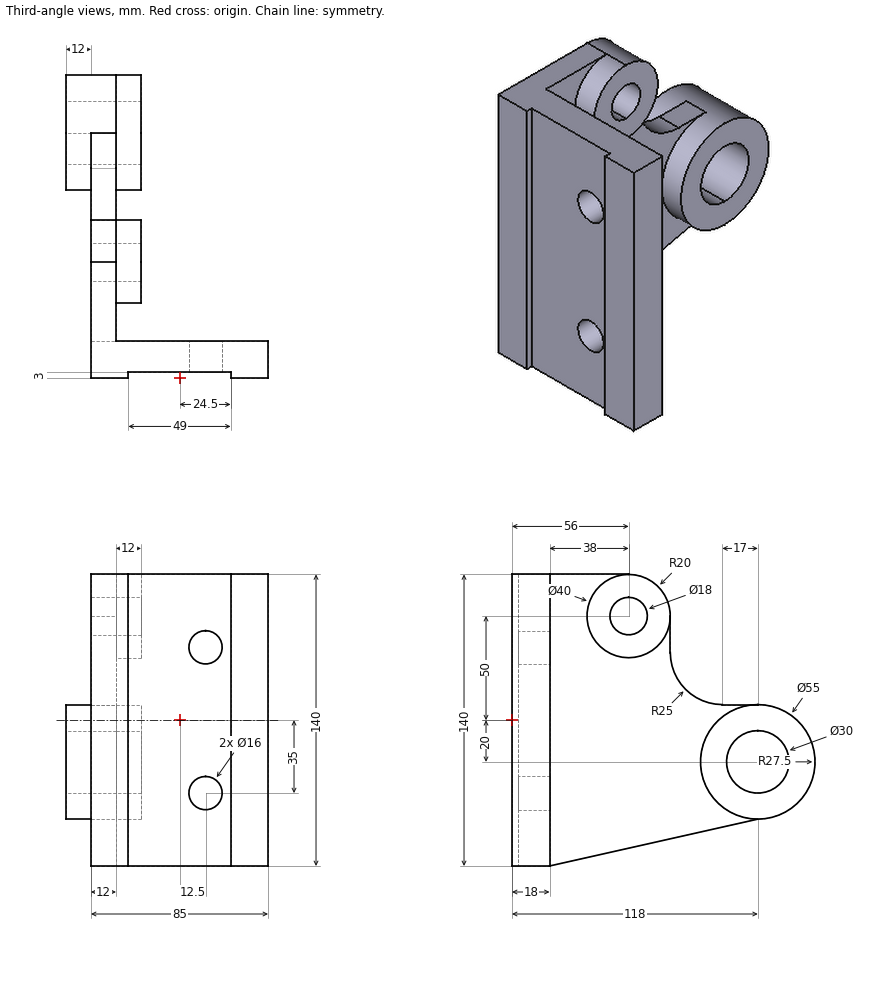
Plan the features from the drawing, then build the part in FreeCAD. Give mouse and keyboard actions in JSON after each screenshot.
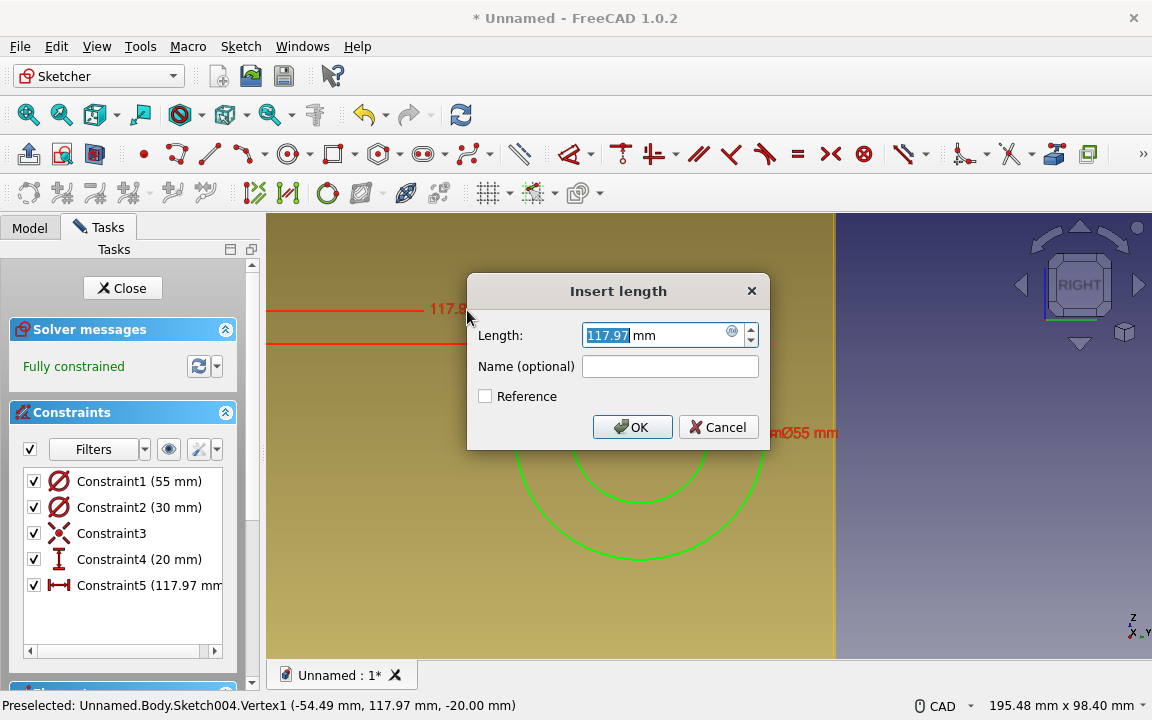
{"action": "type", "text": "118"}
{"action": "key", "text": "Return"}
{"action": "key", "text": "Escape"}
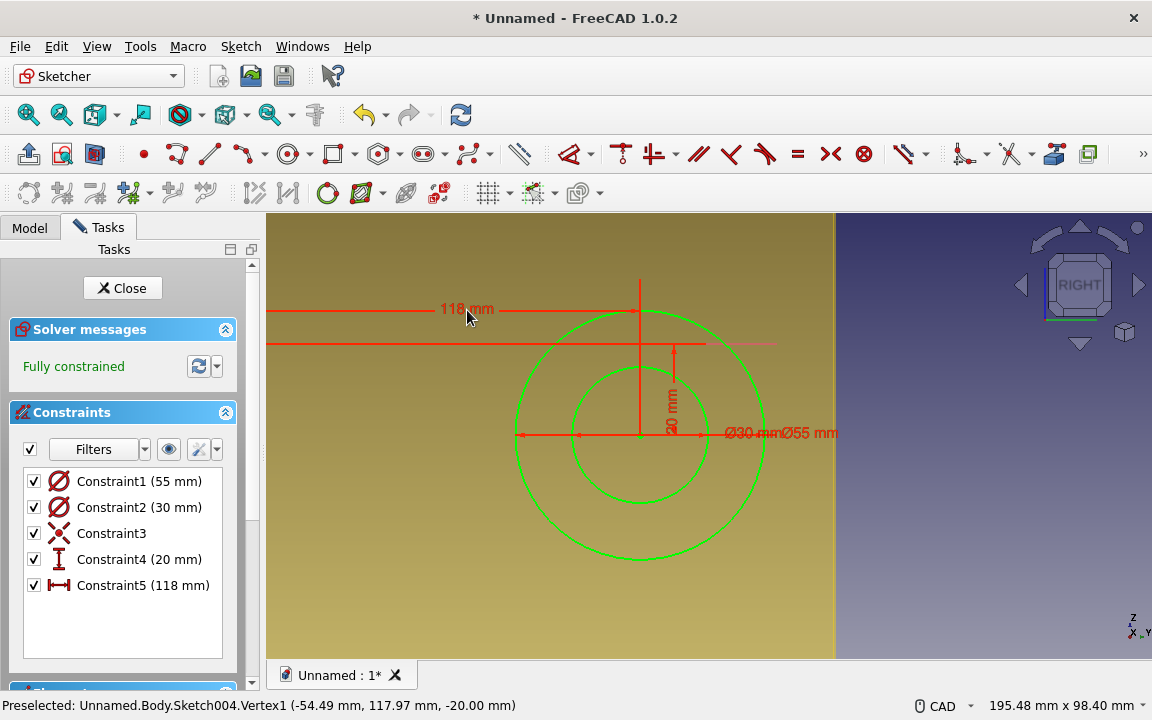
{"action": "left_click", "coordinate": [123, 288]}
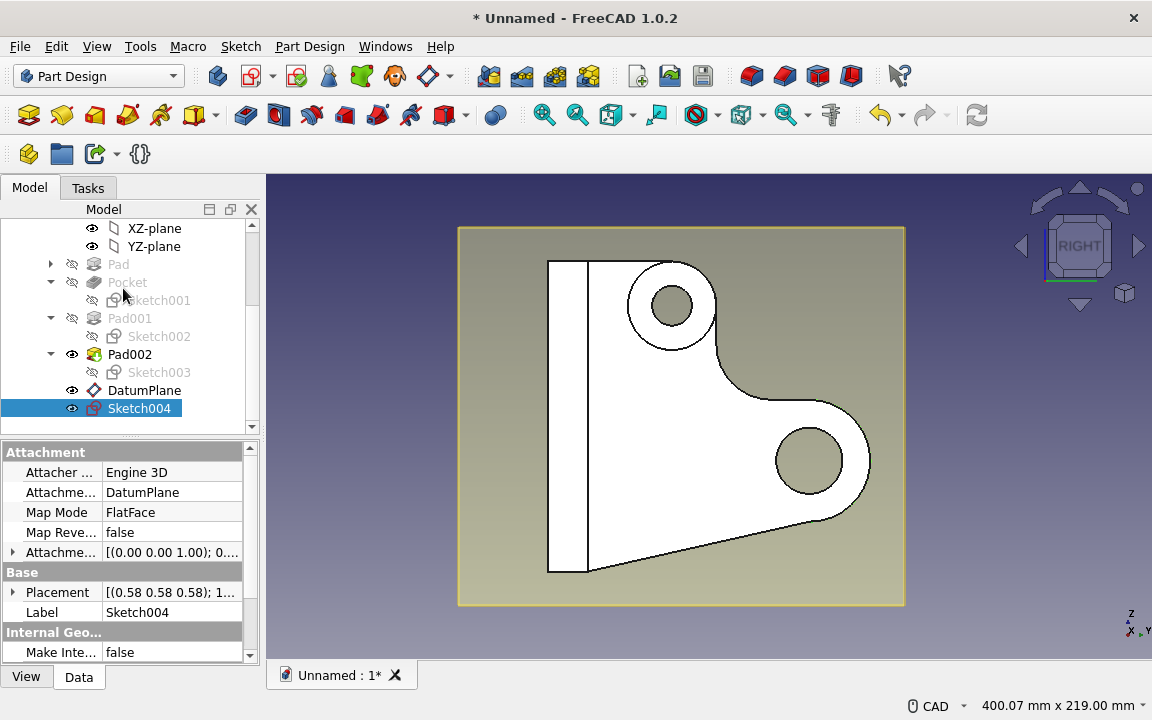
{"action": "left_click", "coordinate": [29, 116]}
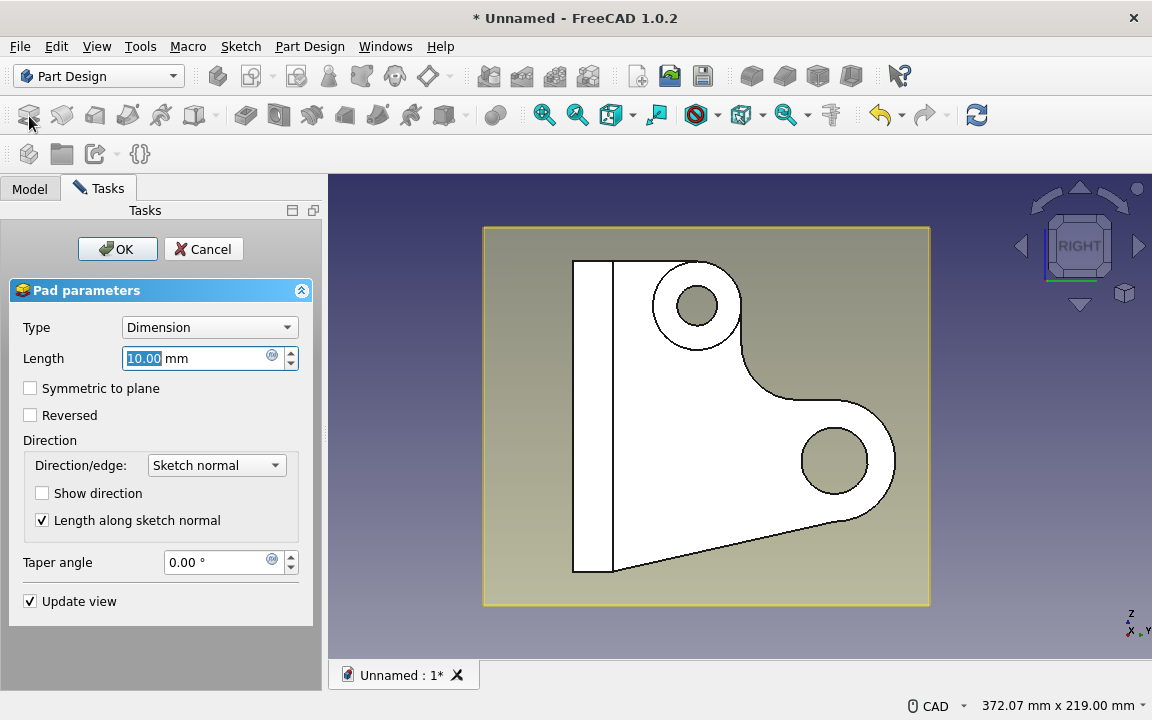
{"action": "type", "text": "12"}
{"action": "key", "text": "Tab"}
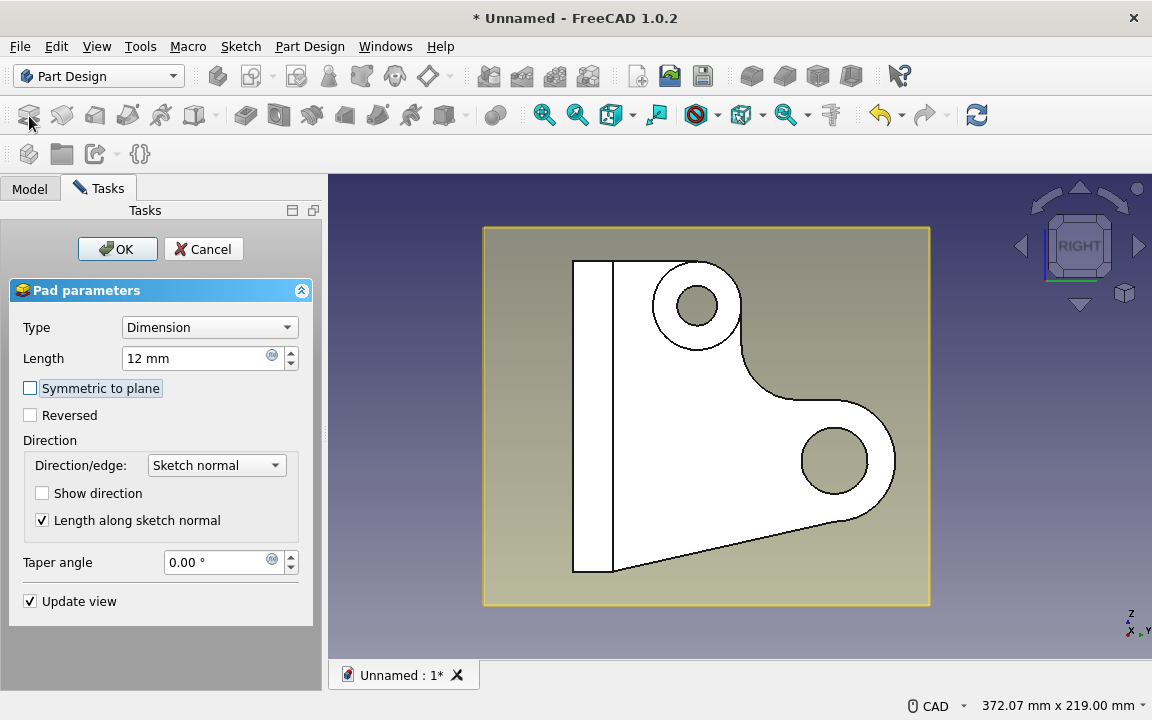
{"action": "left_click", "coordinate": [118, 249]}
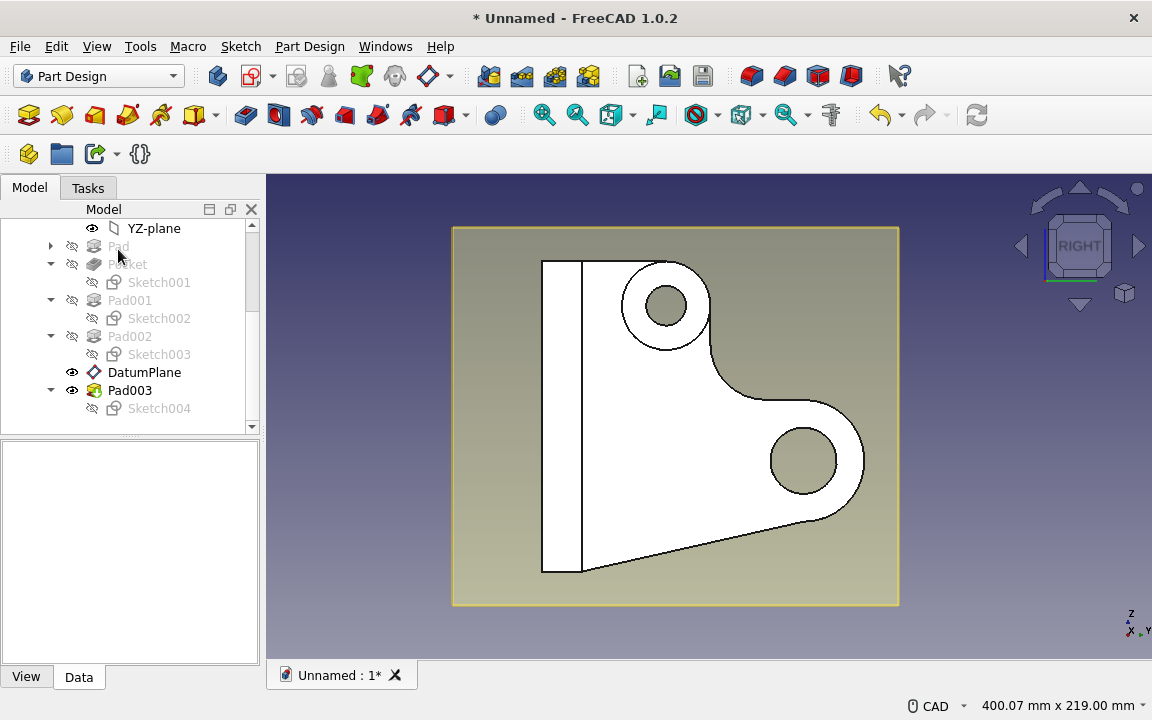
{"action": "left_click", "coordinate": [117, 372]}
{"action": "key", "text": "space"}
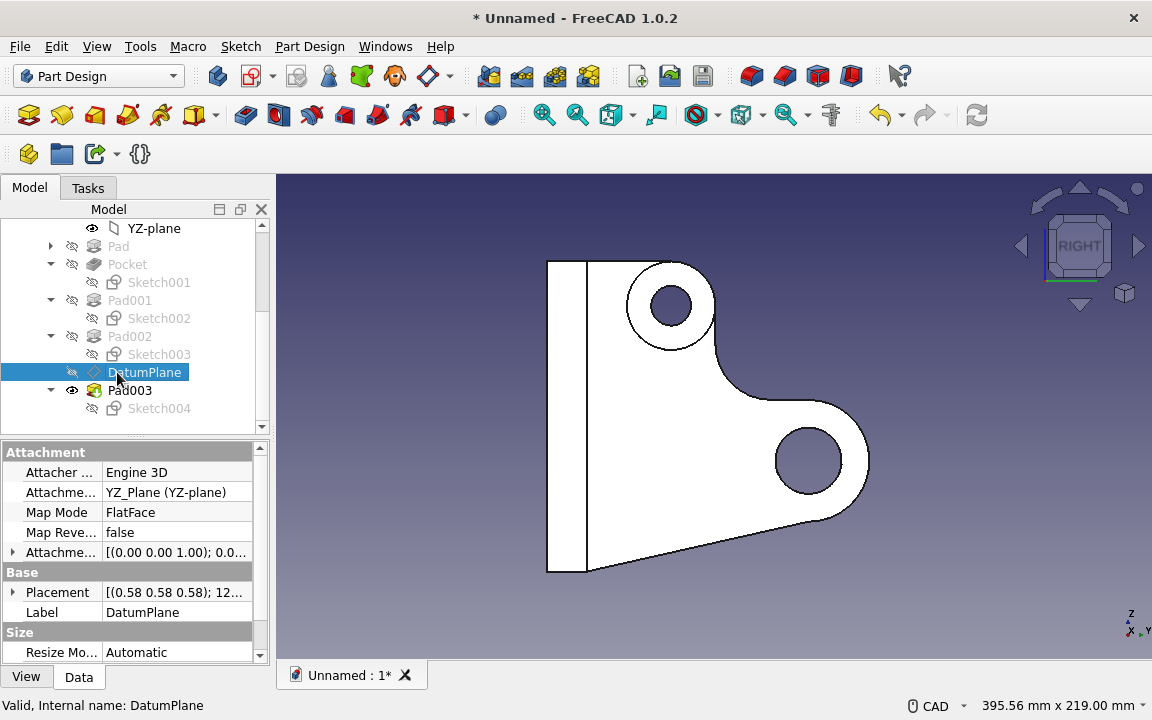
{"action": "left_click", "coordinate": [688, 460]}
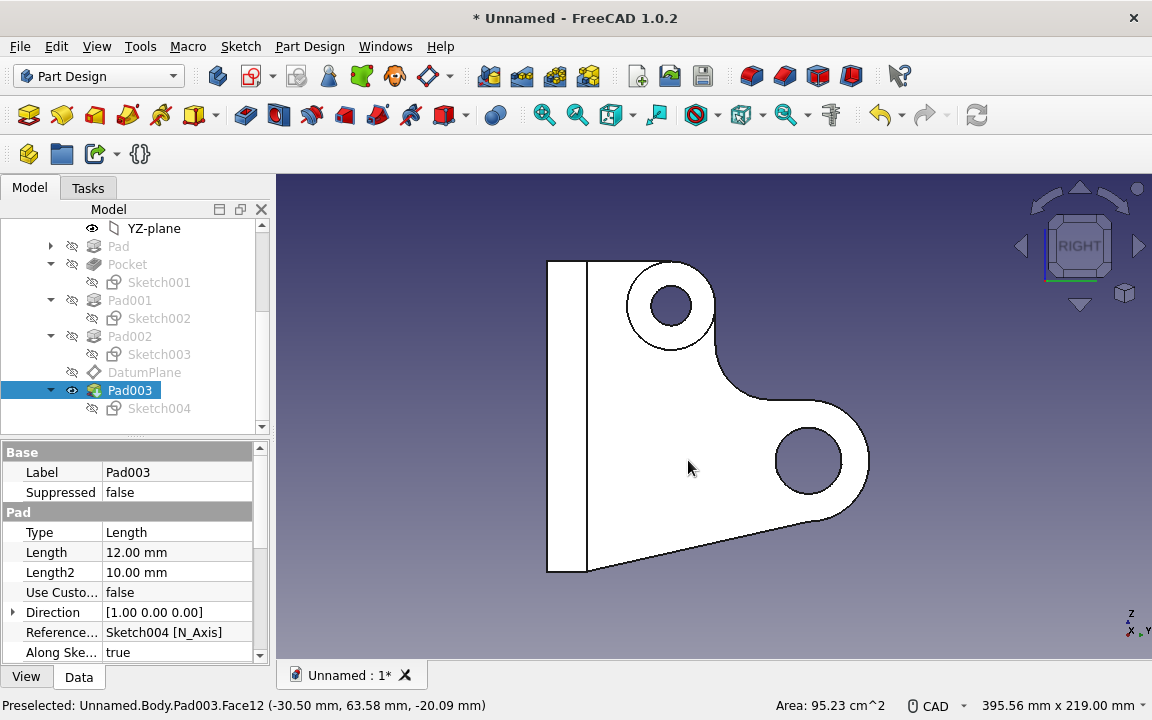
{"action": "left_click", "coordinate": [250, 76]}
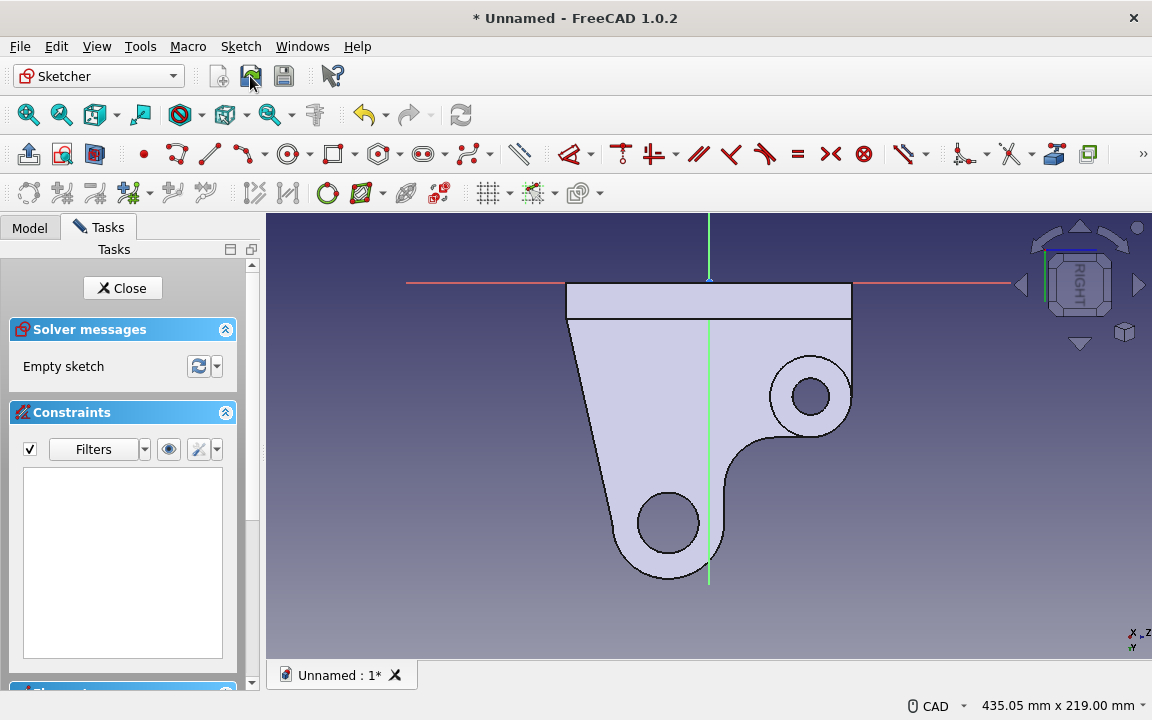
{"action": "scroll", "coordinate": [691, 594], "scroll_direction": "up", "scroll_amount": 4}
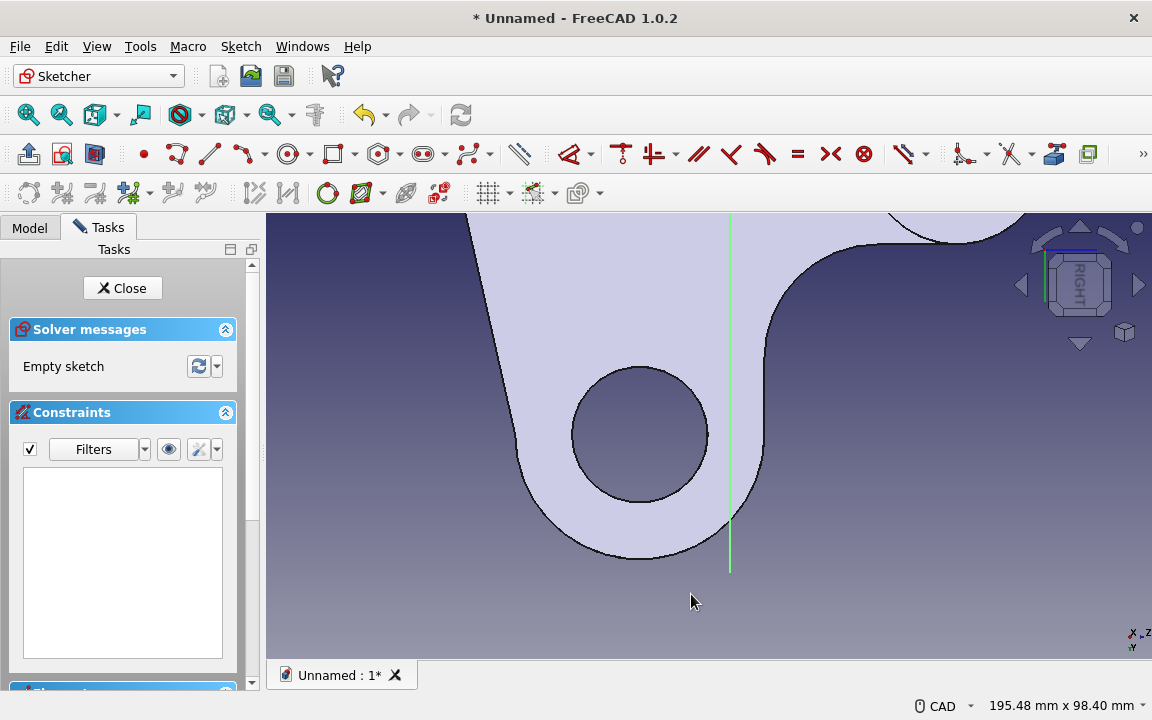
{"action": "key", "text": "g c"}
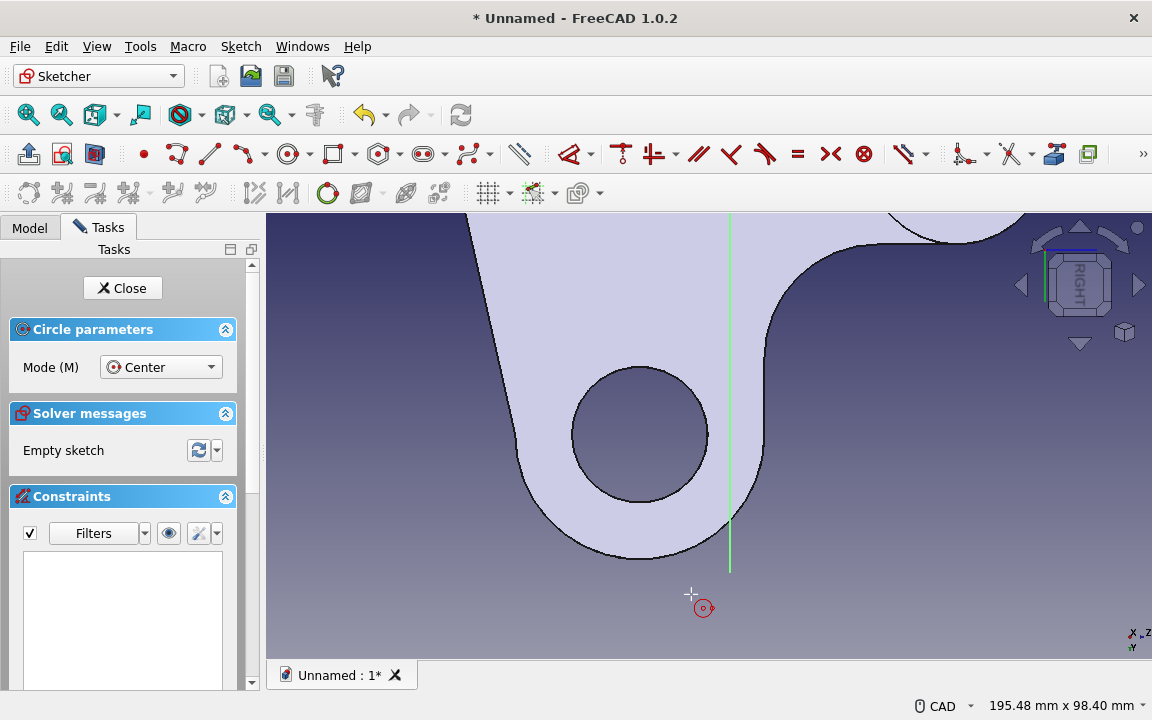
{"action": "left_click", "coordinate": [640, 435]}
{"action": "mouse_move", "coordinate": [552, 347]}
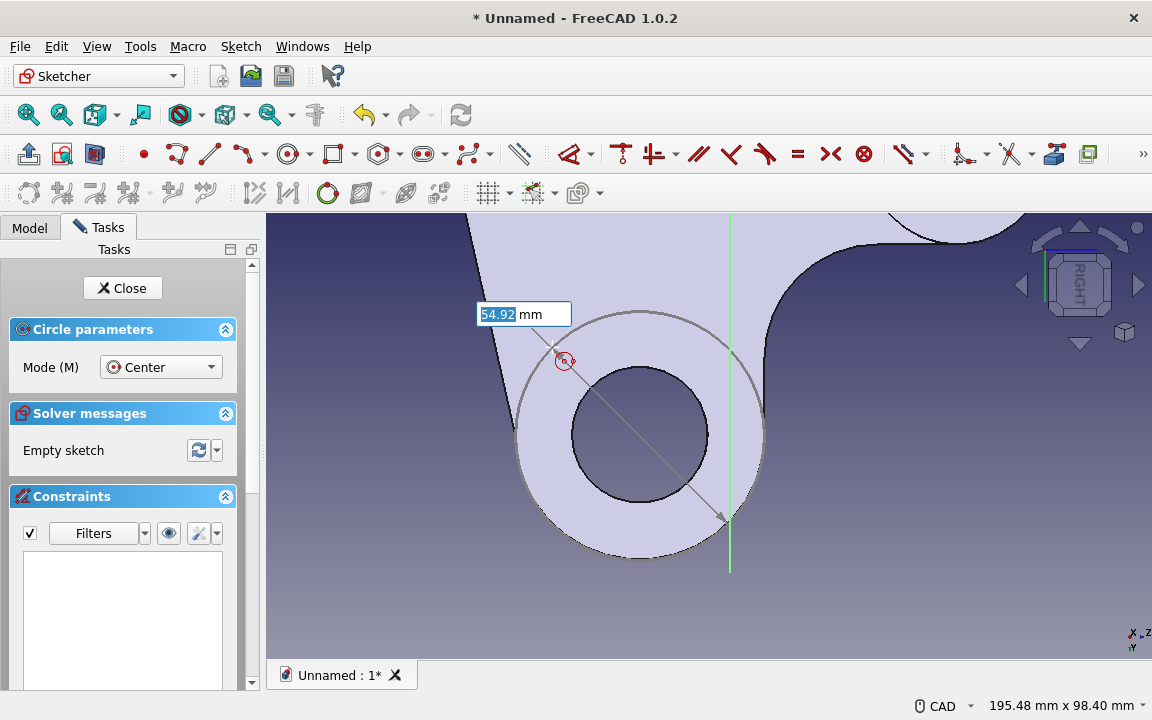
{"action": "type", "text": "55"}
{"action": "key", "text": "Return"}